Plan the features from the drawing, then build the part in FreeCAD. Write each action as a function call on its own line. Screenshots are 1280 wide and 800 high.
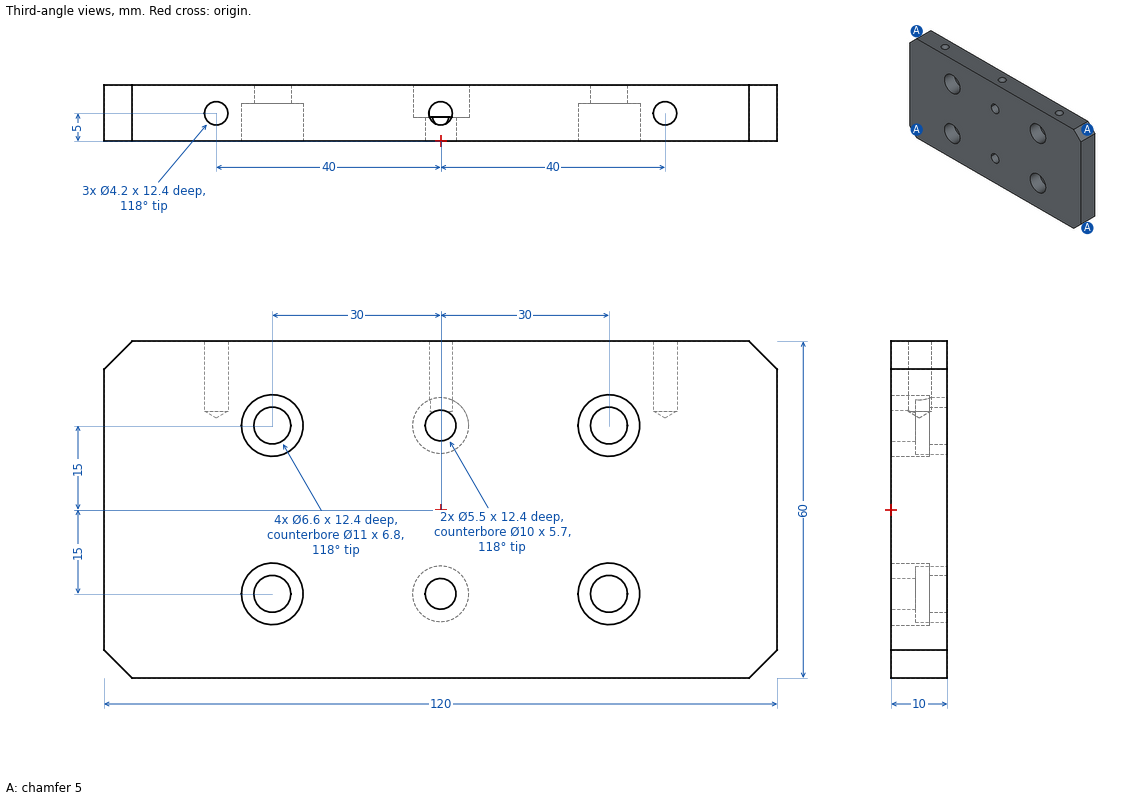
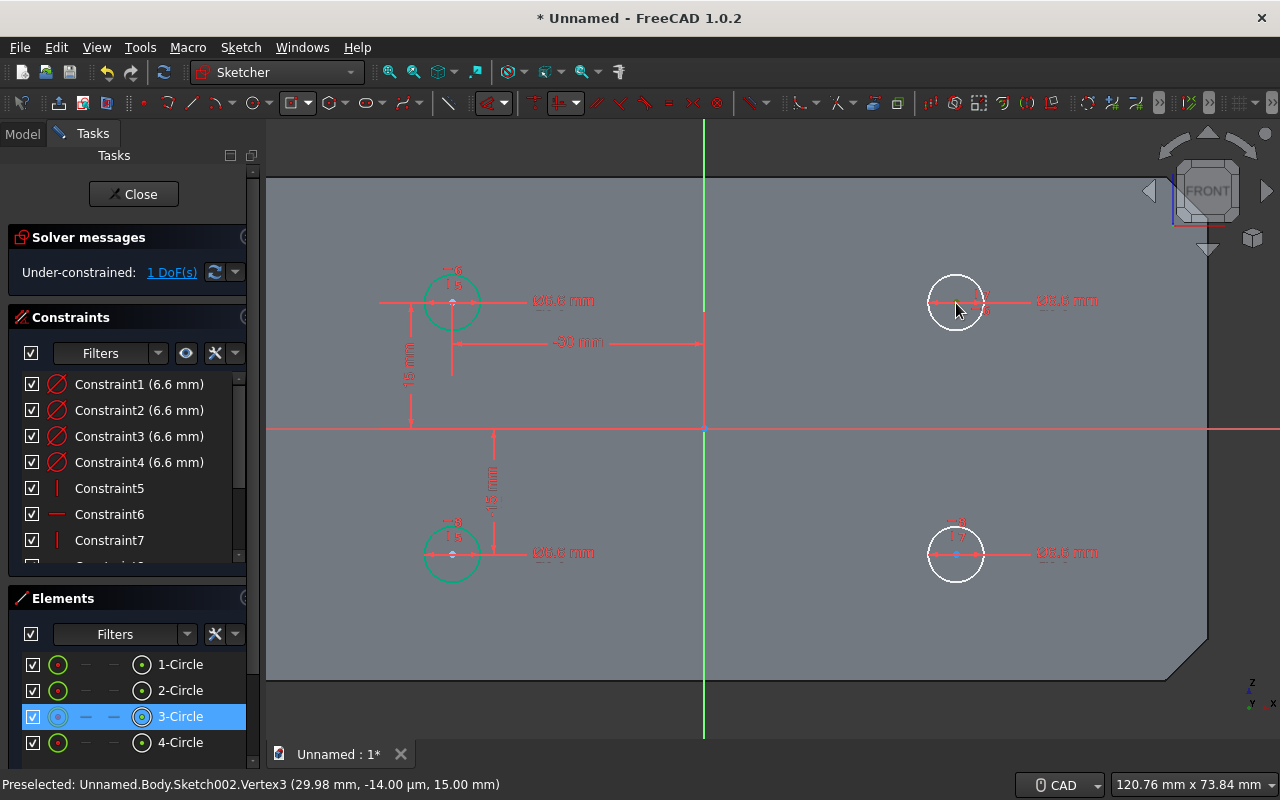
key(l)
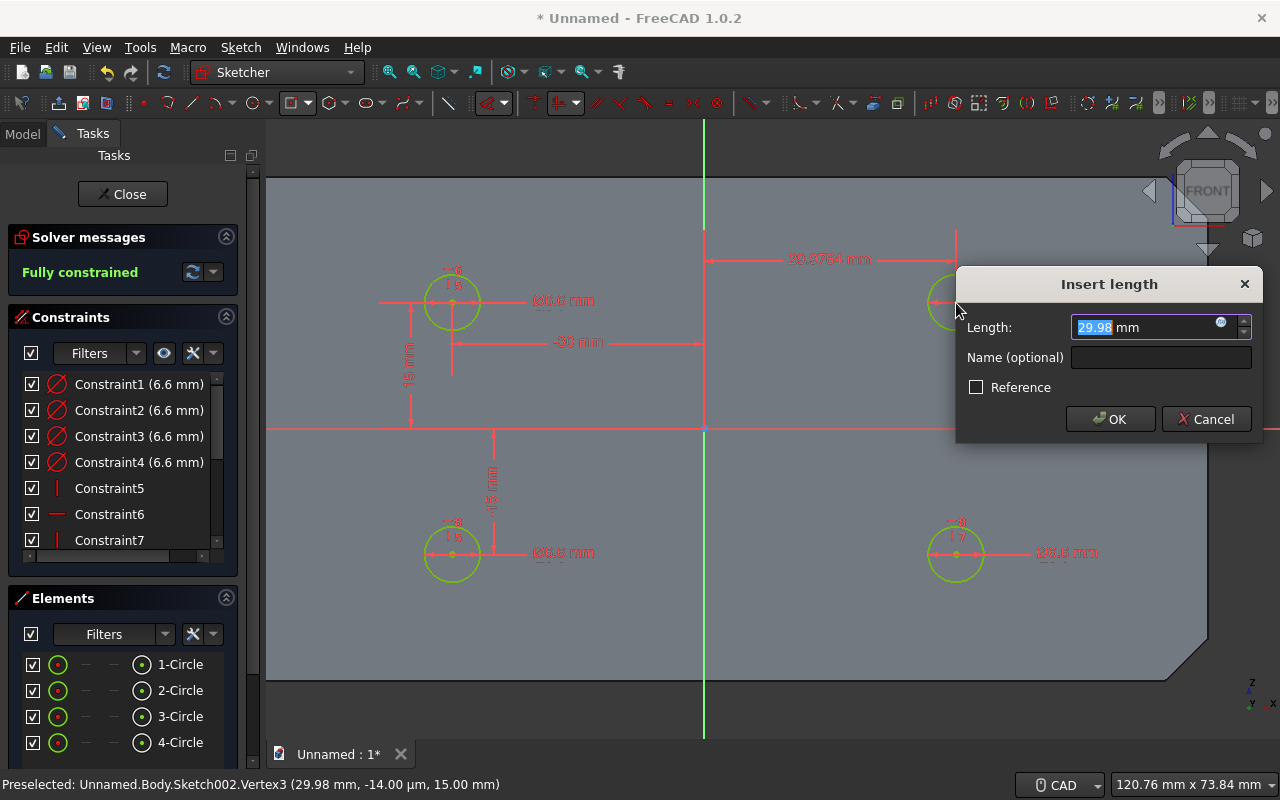
text(30)
key(Return)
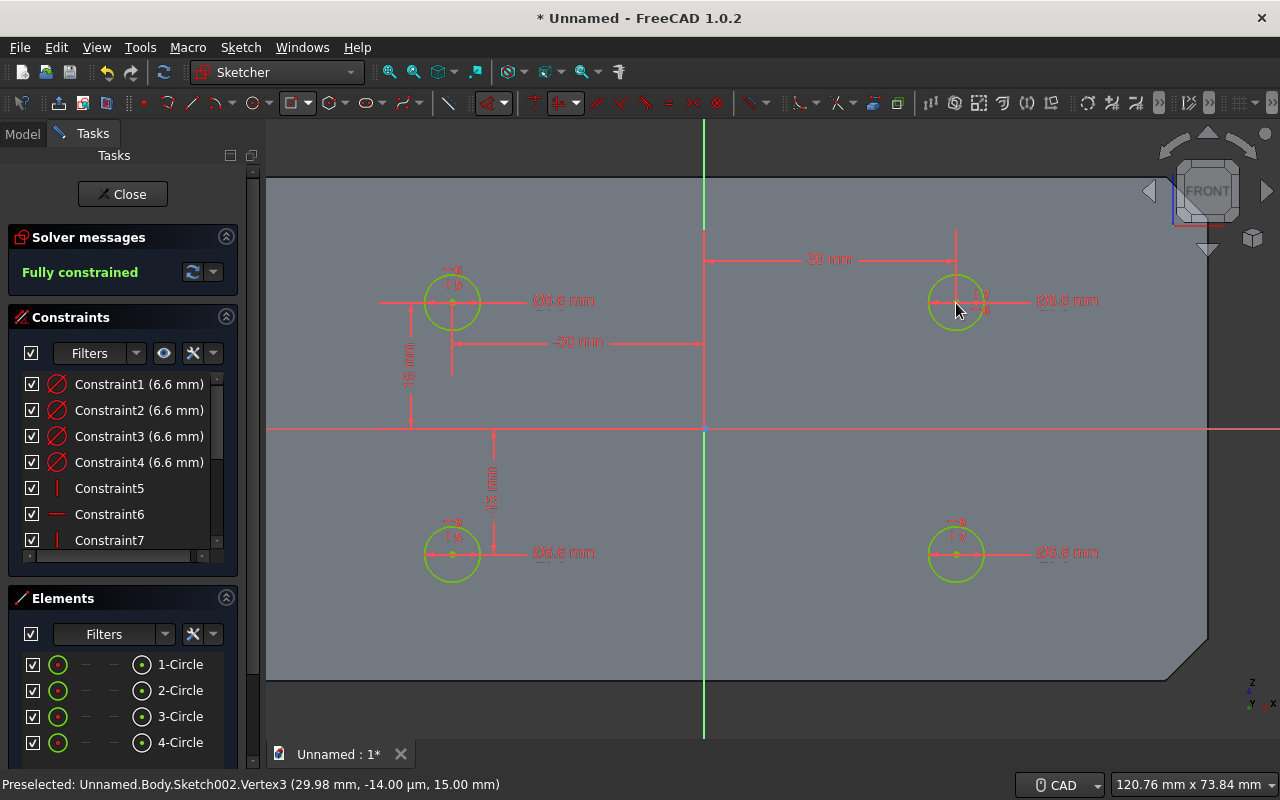
click(123, 194)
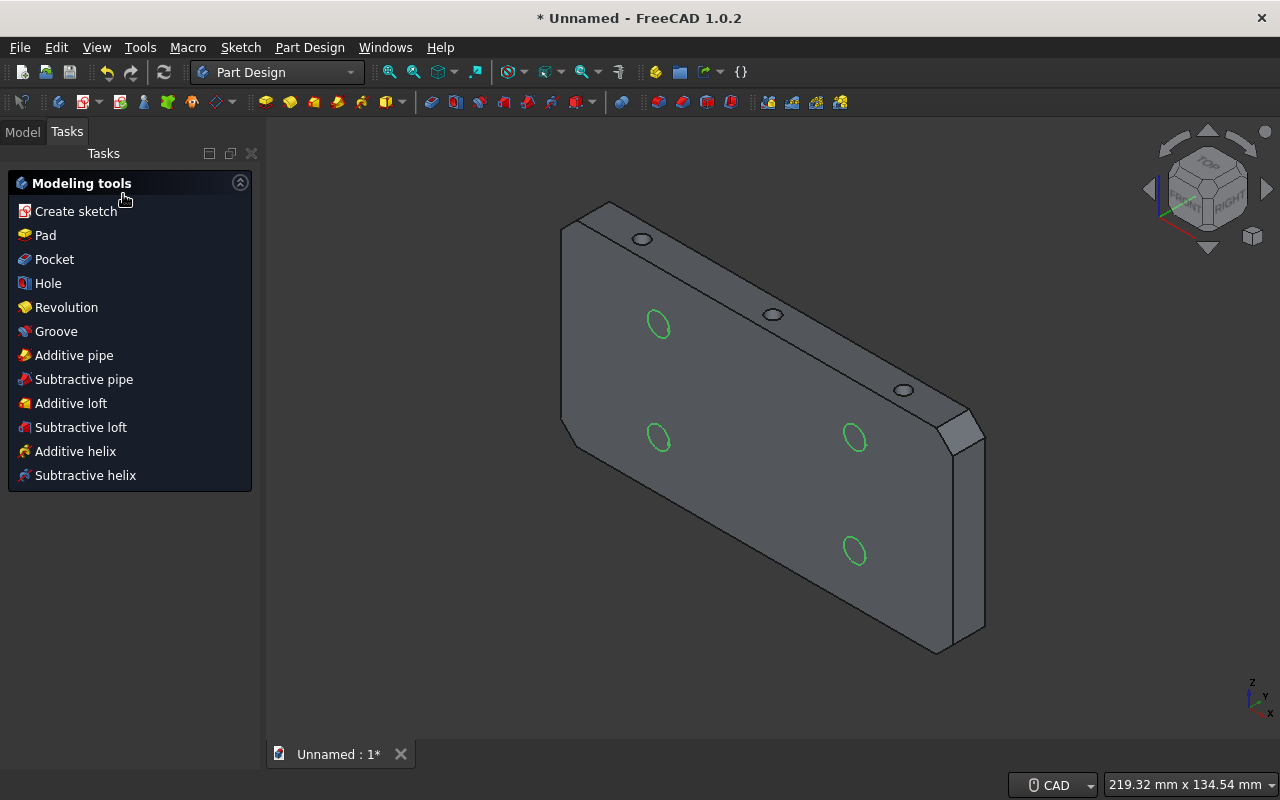
click(456, 102)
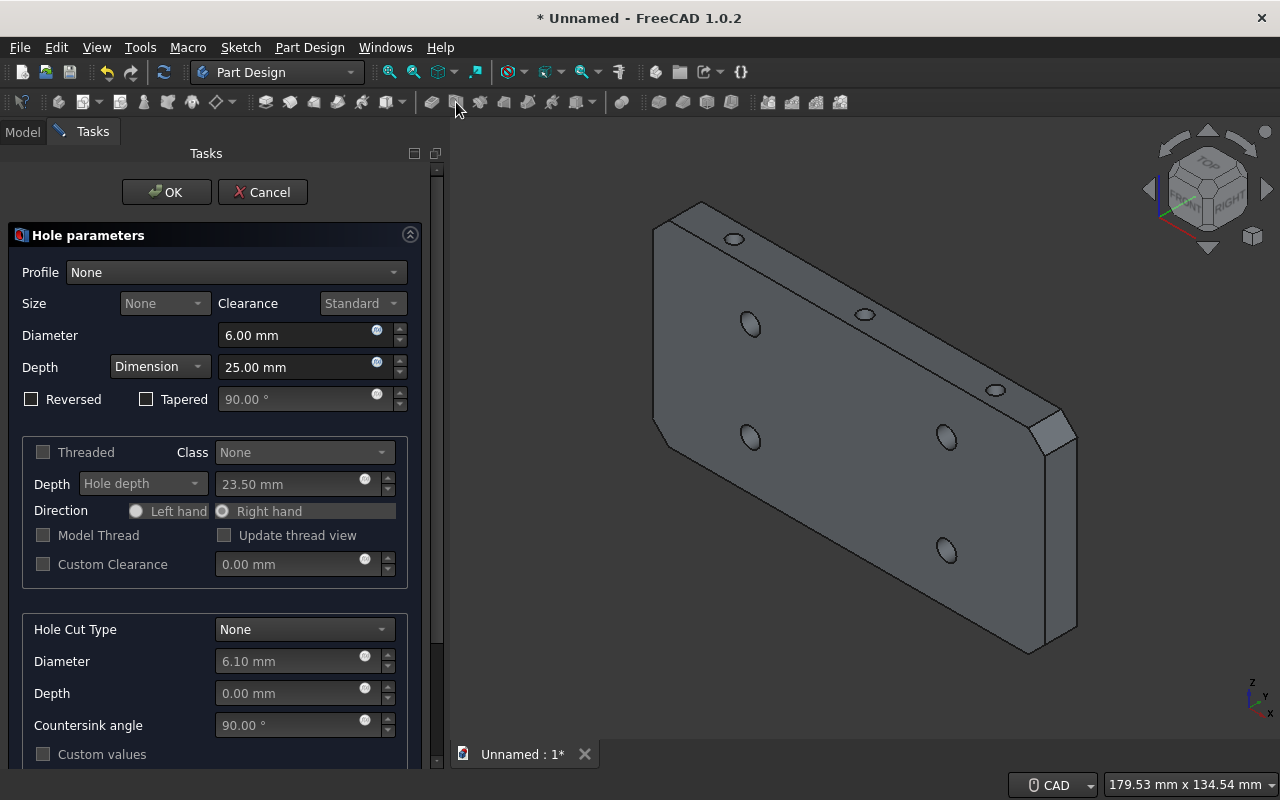
triple_click(305, 335)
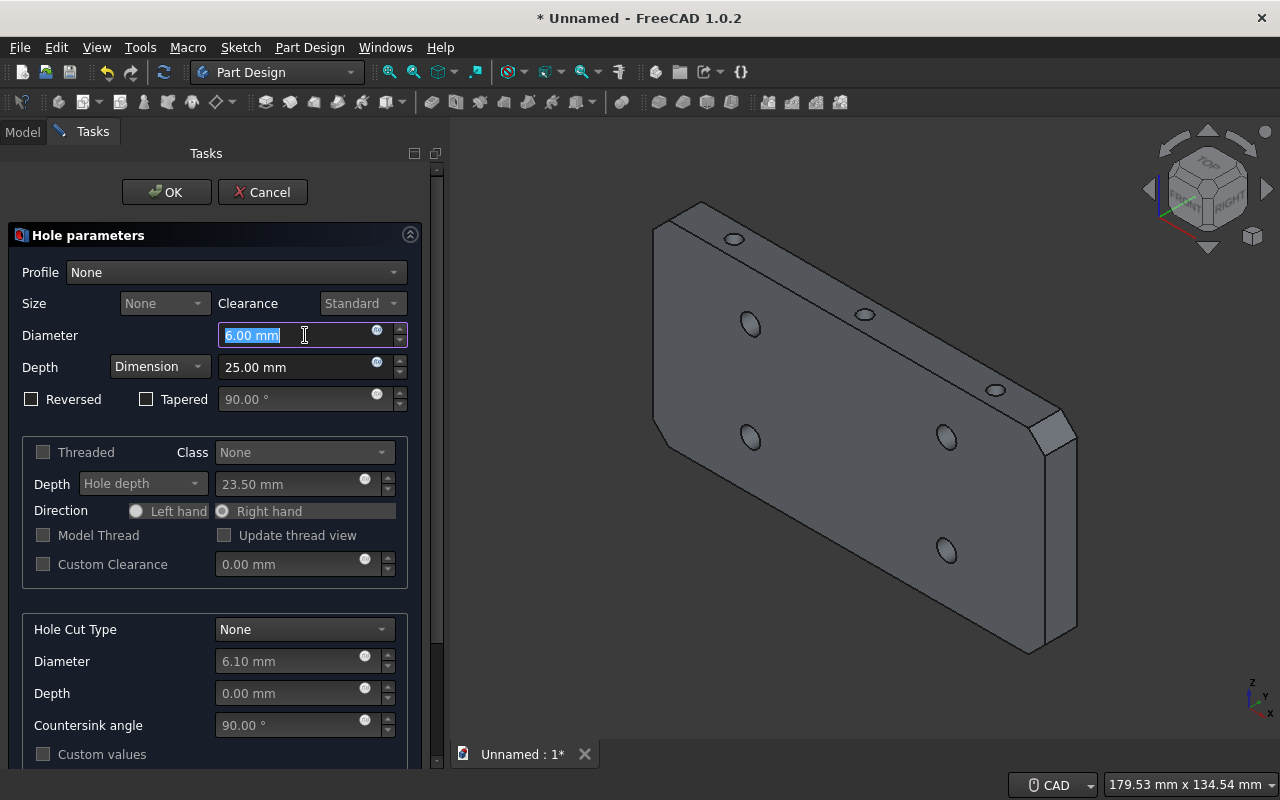
text(6.6)
key(Tab)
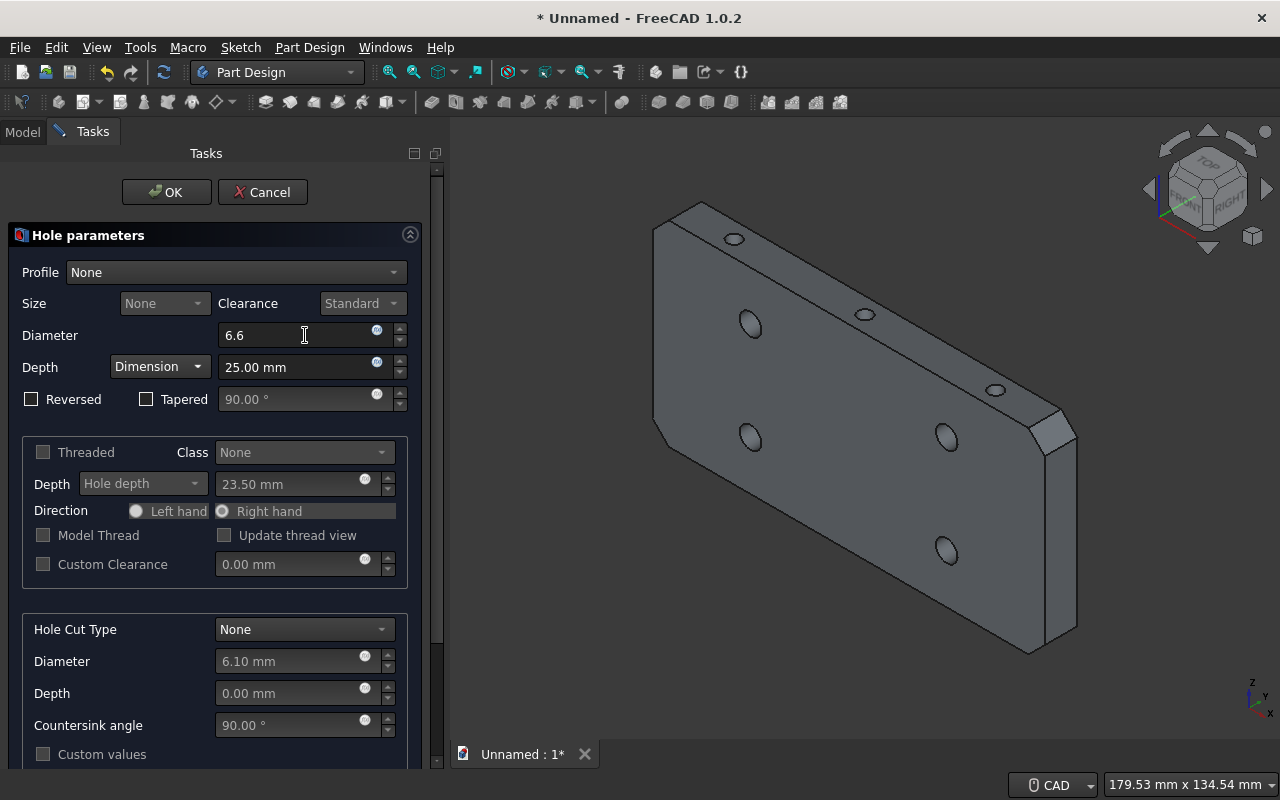
triple_click(305, 367)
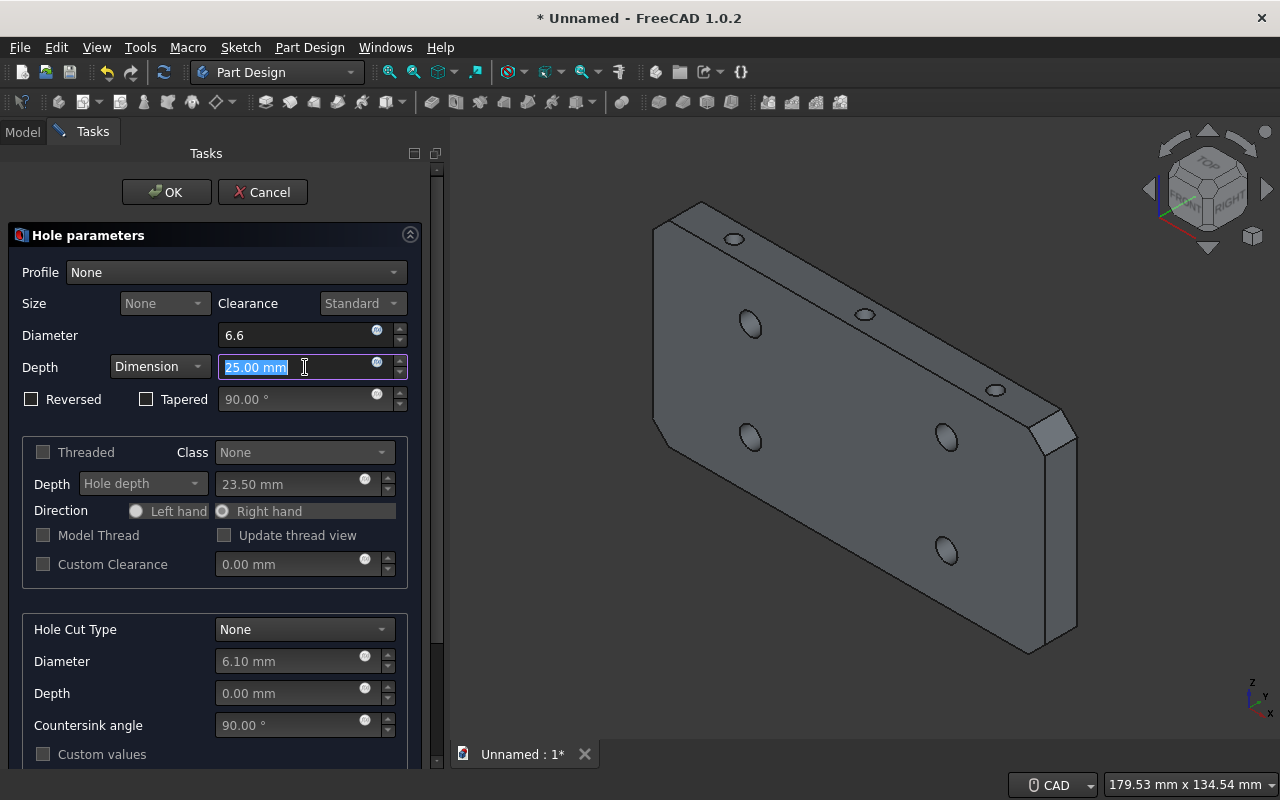
text(12.4)
key(Tab)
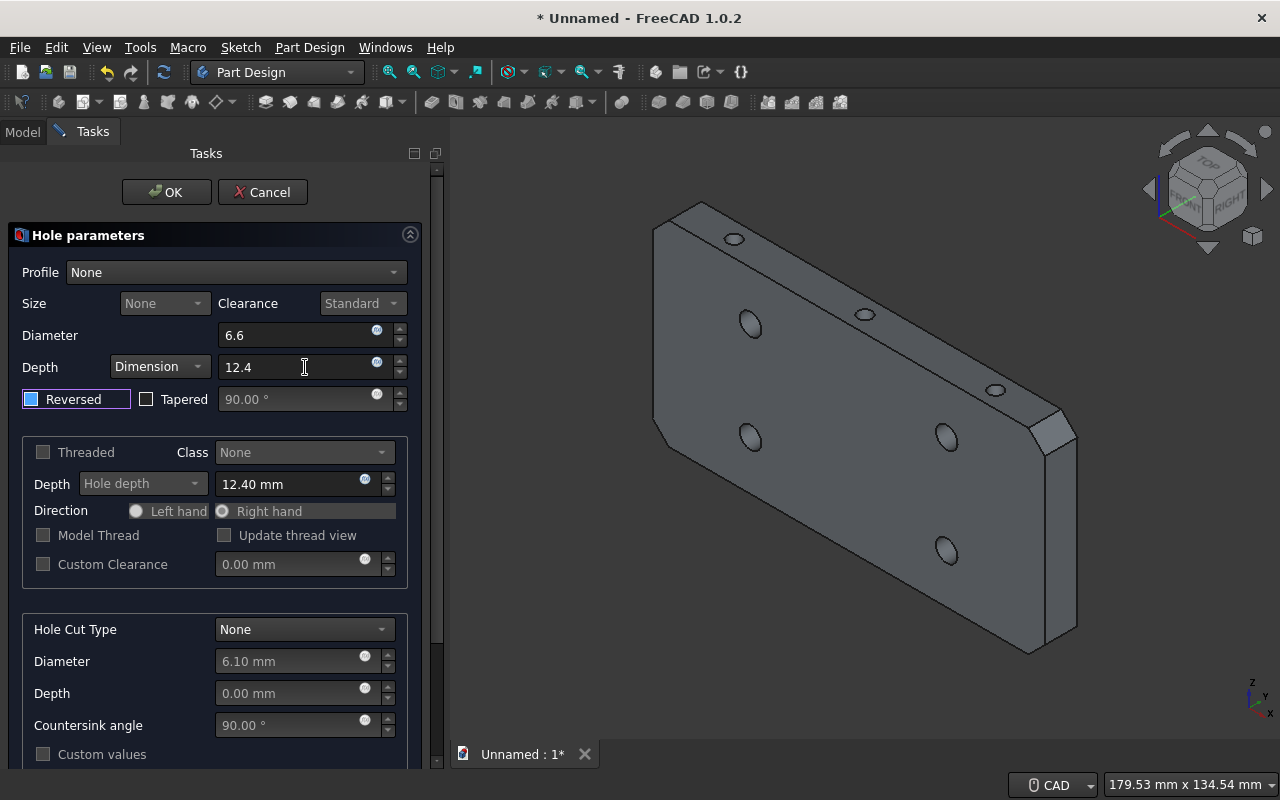
click(306, 630)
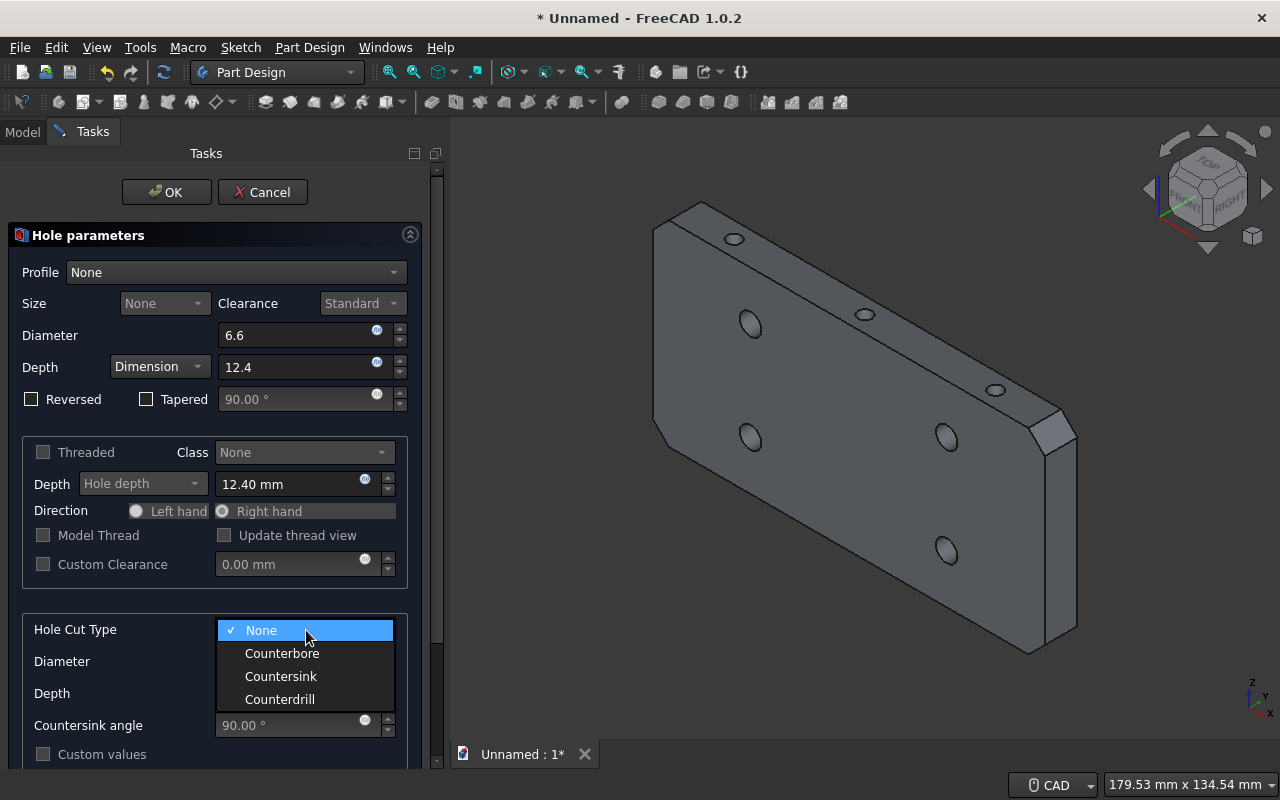
click(304, 654)